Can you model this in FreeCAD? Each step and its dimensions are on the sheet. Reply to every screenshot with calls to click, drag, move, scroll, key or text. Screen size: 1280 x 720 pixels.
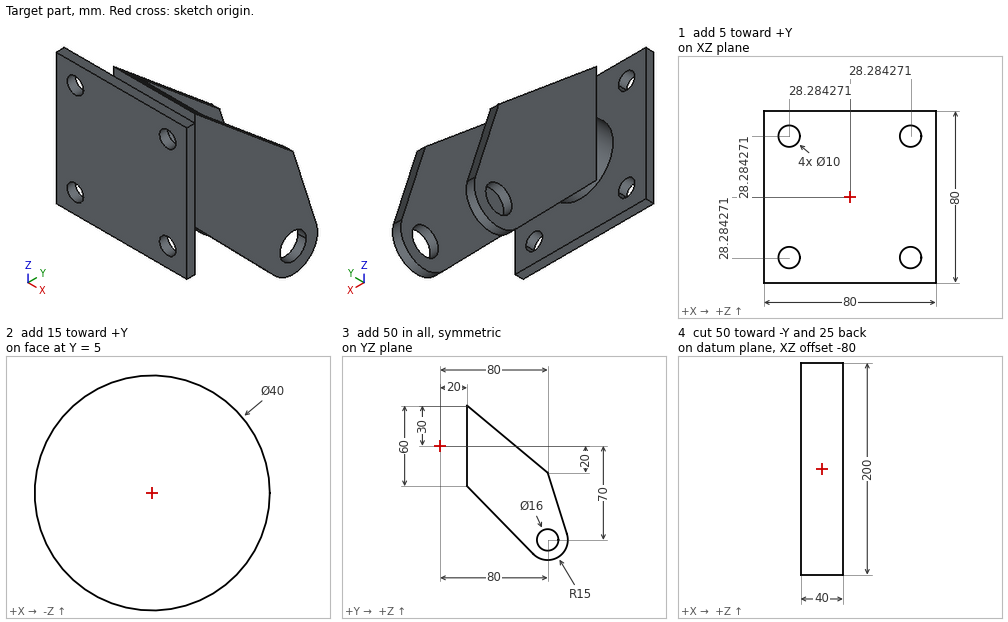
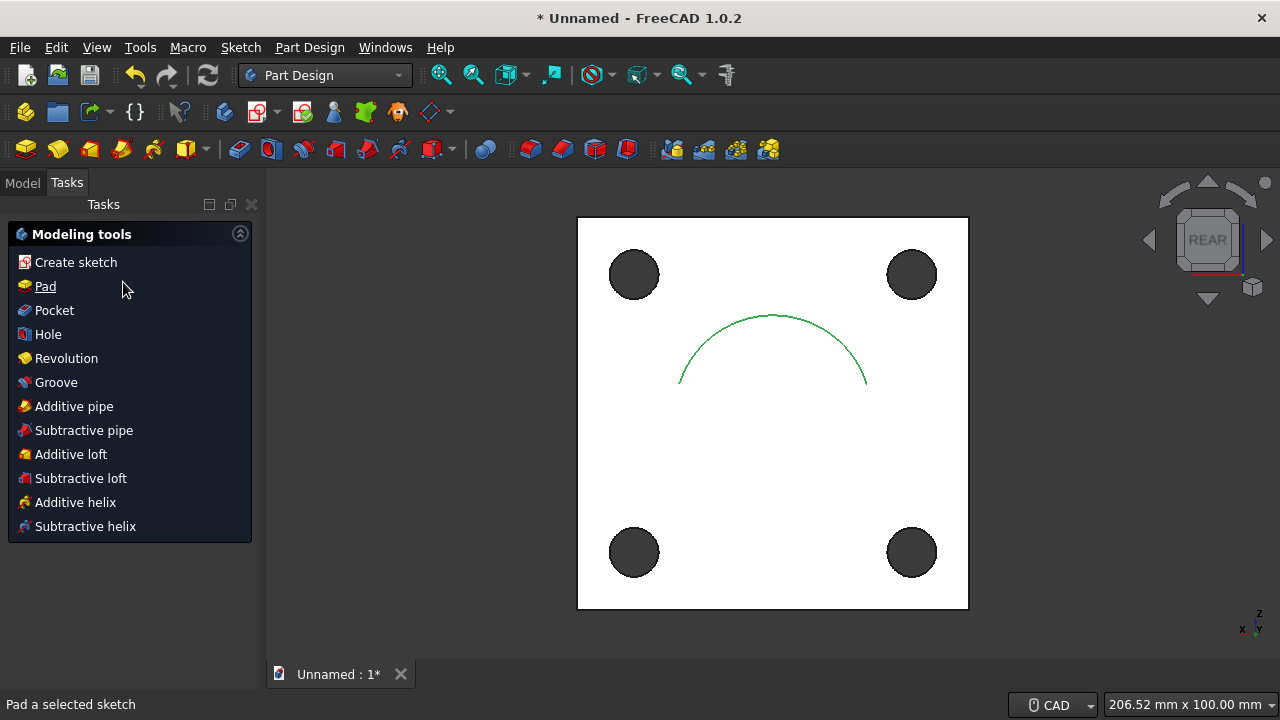
click(26, 150)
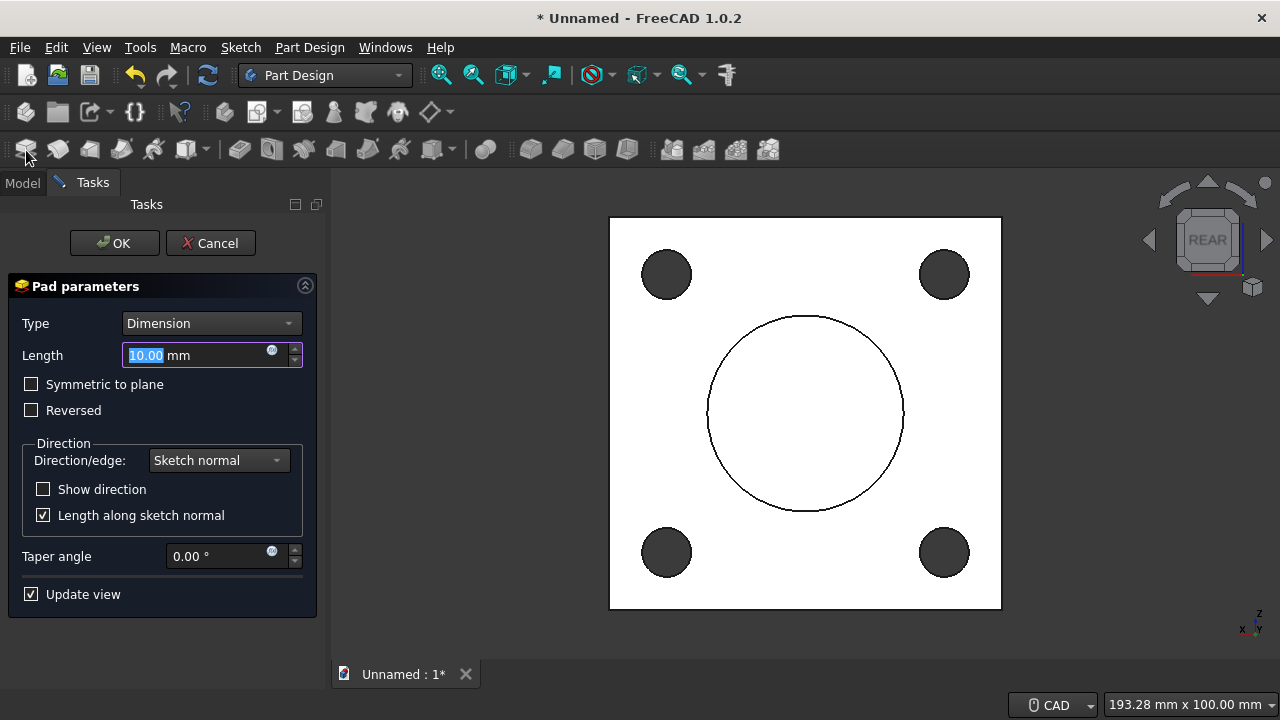
text(15)
key(Tab)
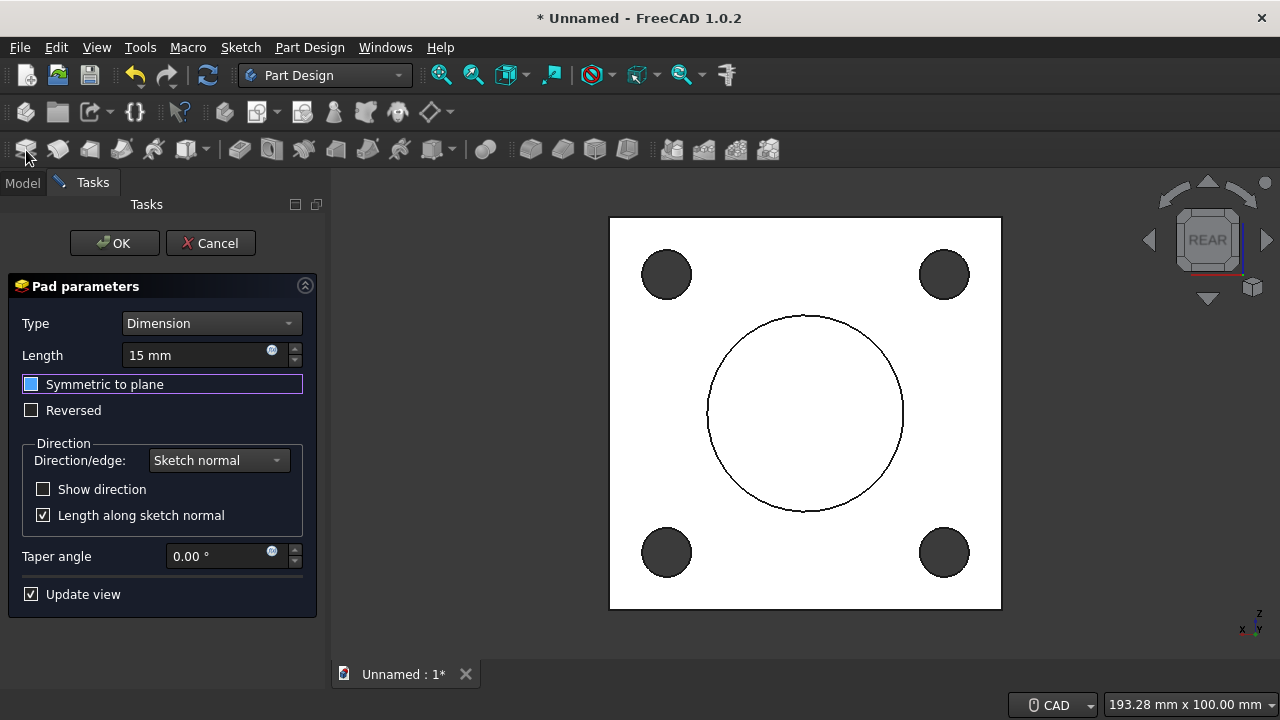
click(115, 243)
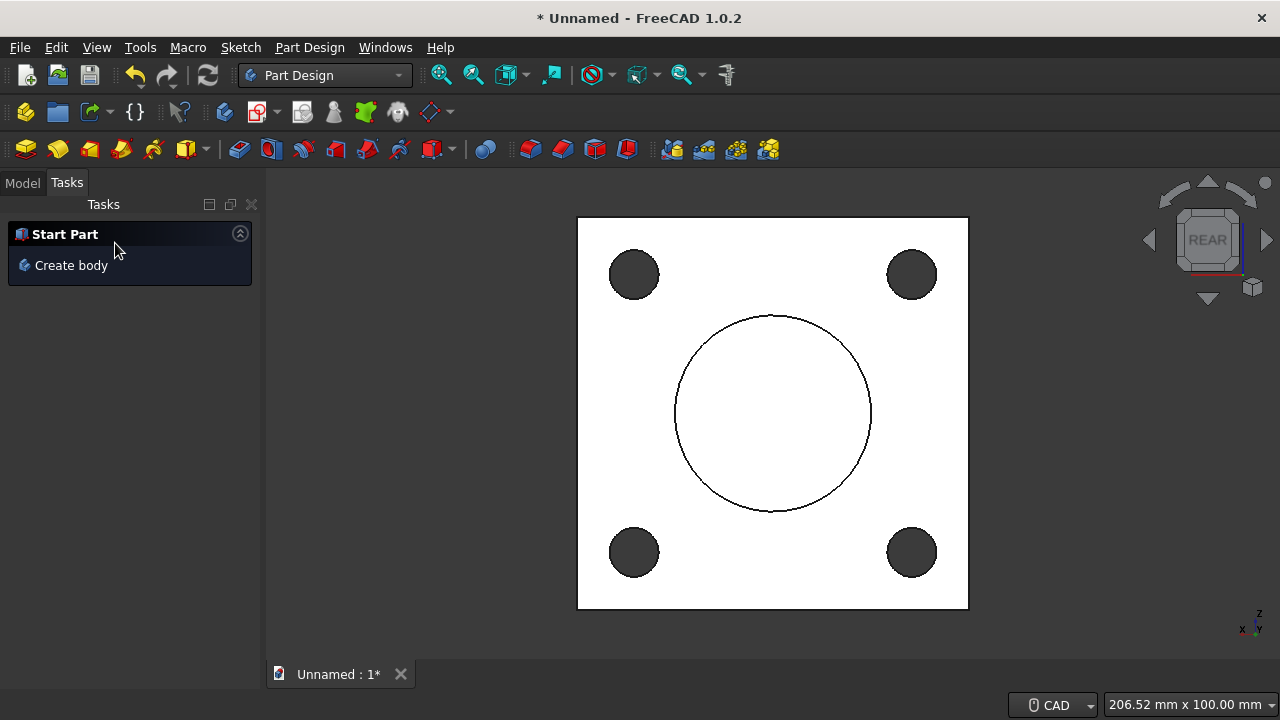
click(258, 112)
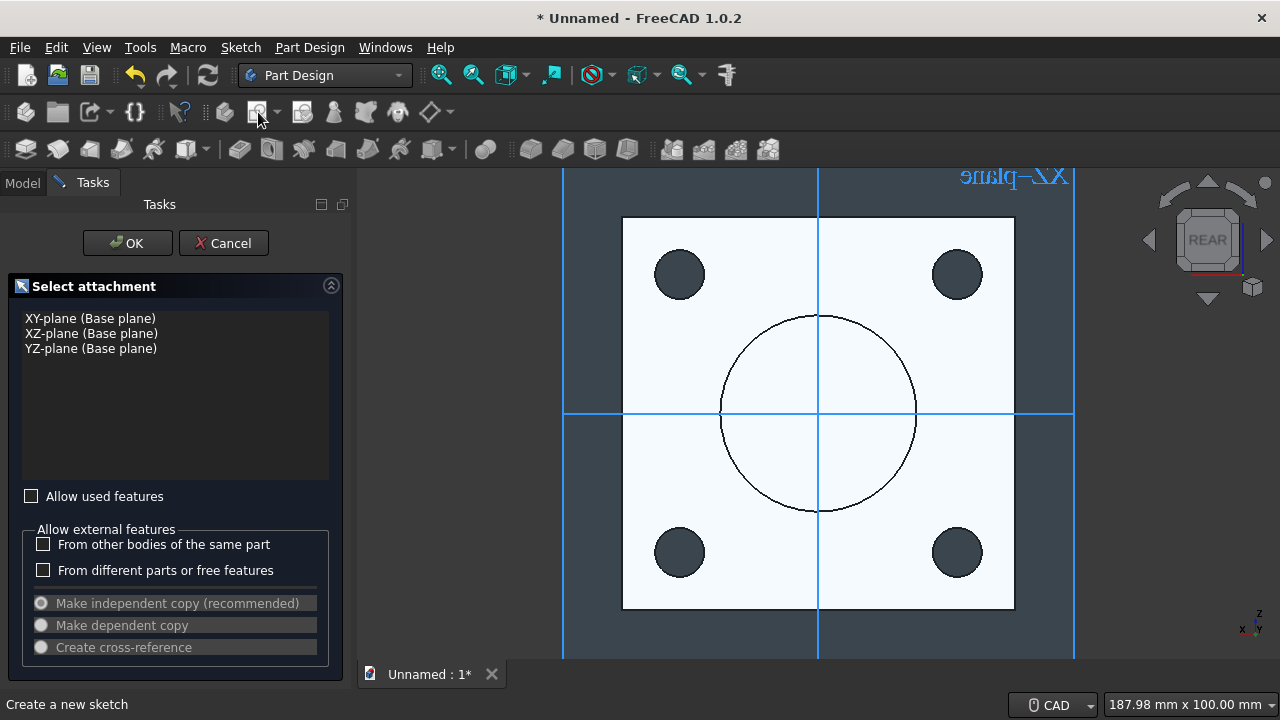
click(82, 348)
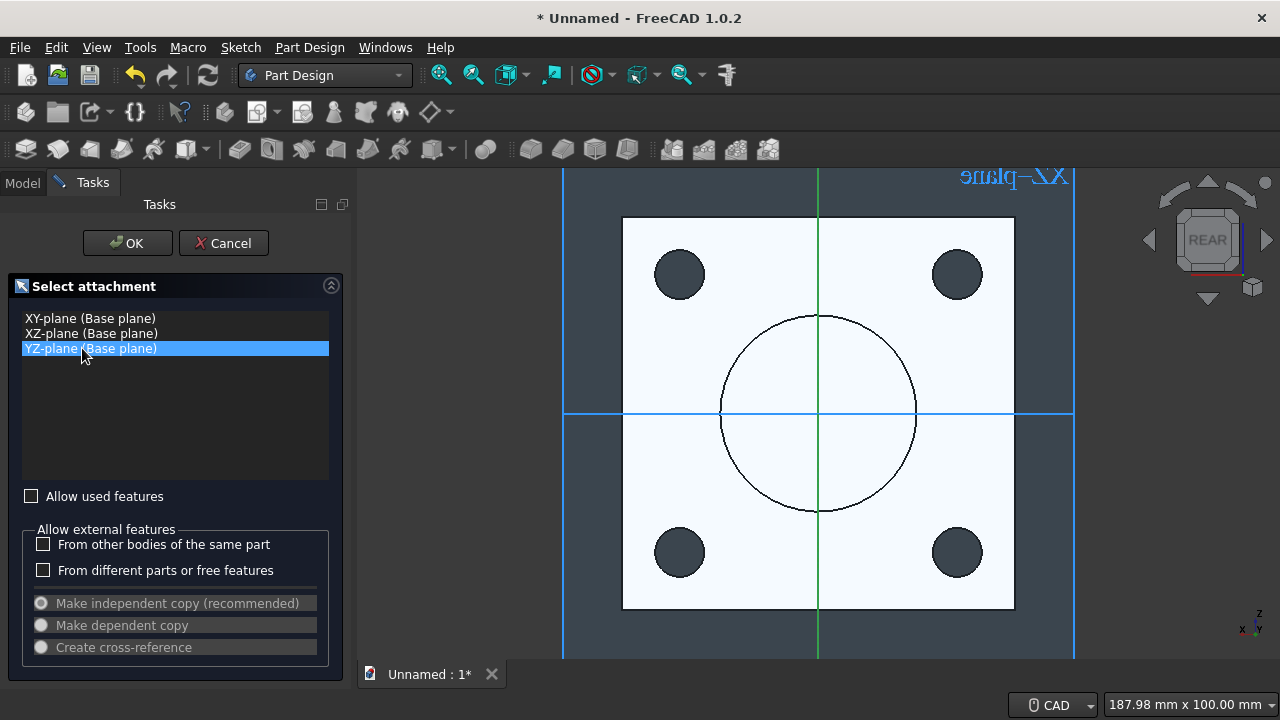
click(128, 243)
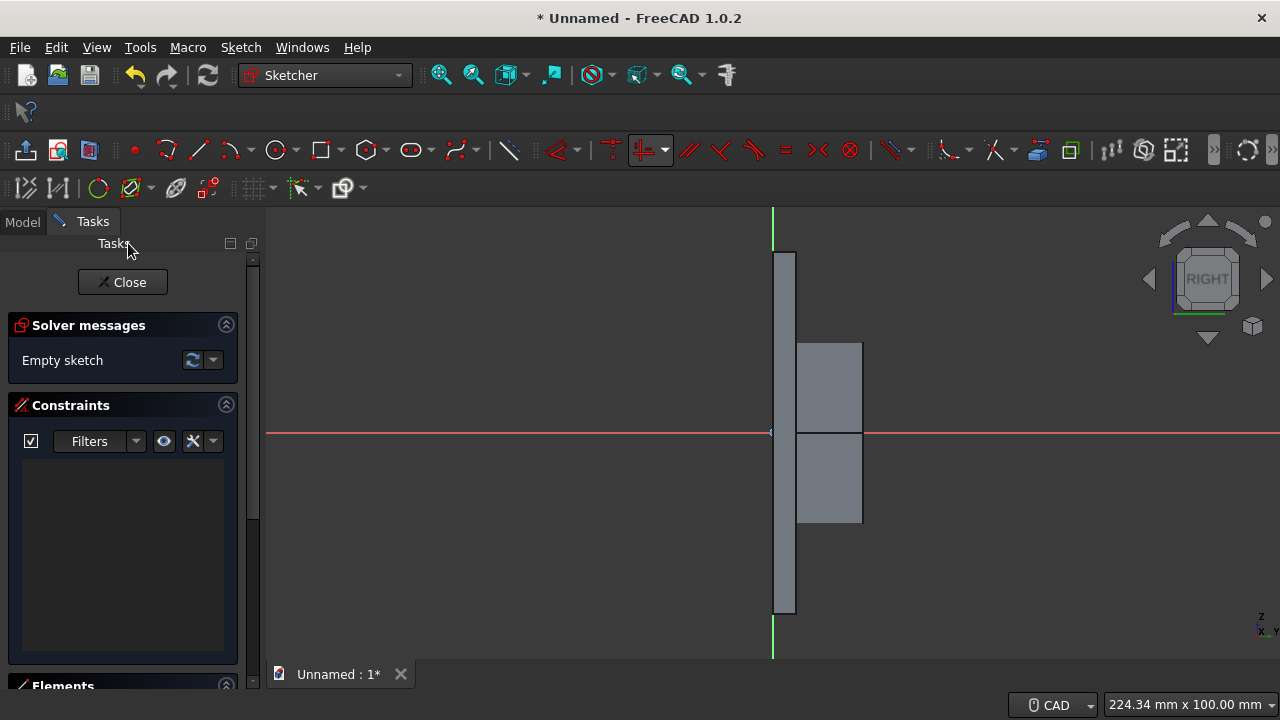
click(90, 150)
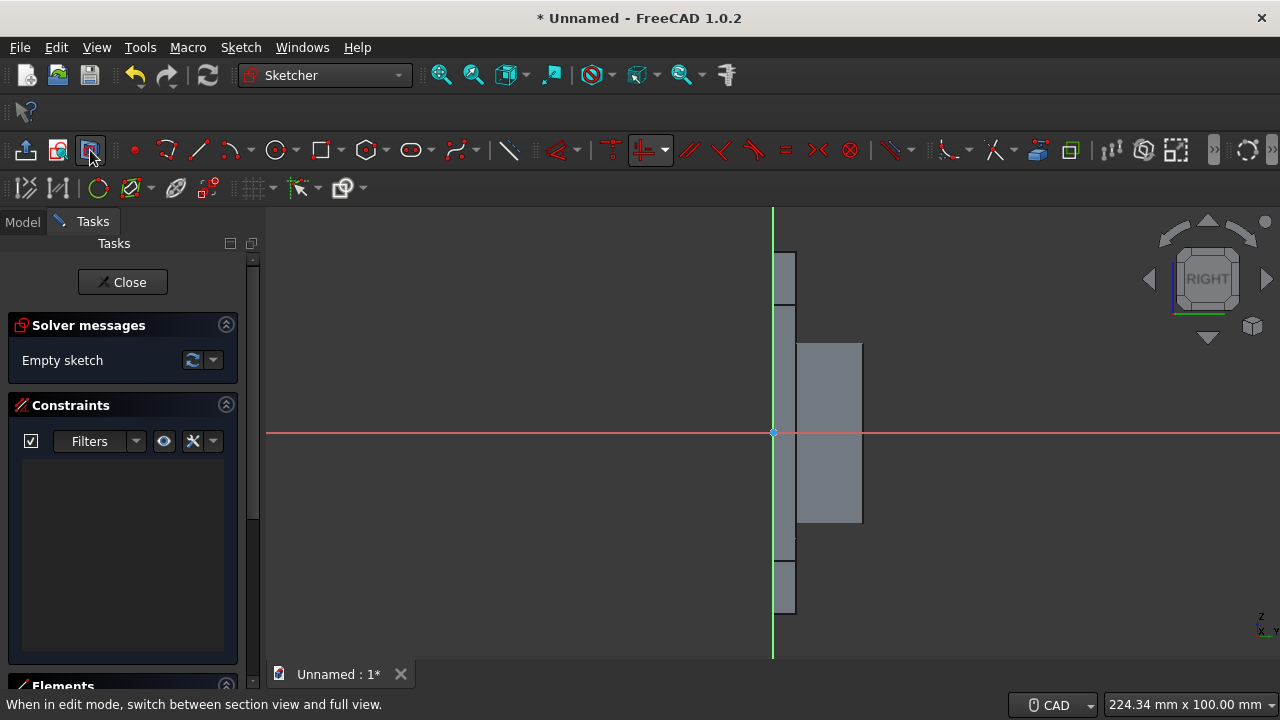
scroll(362, 288, down, 3)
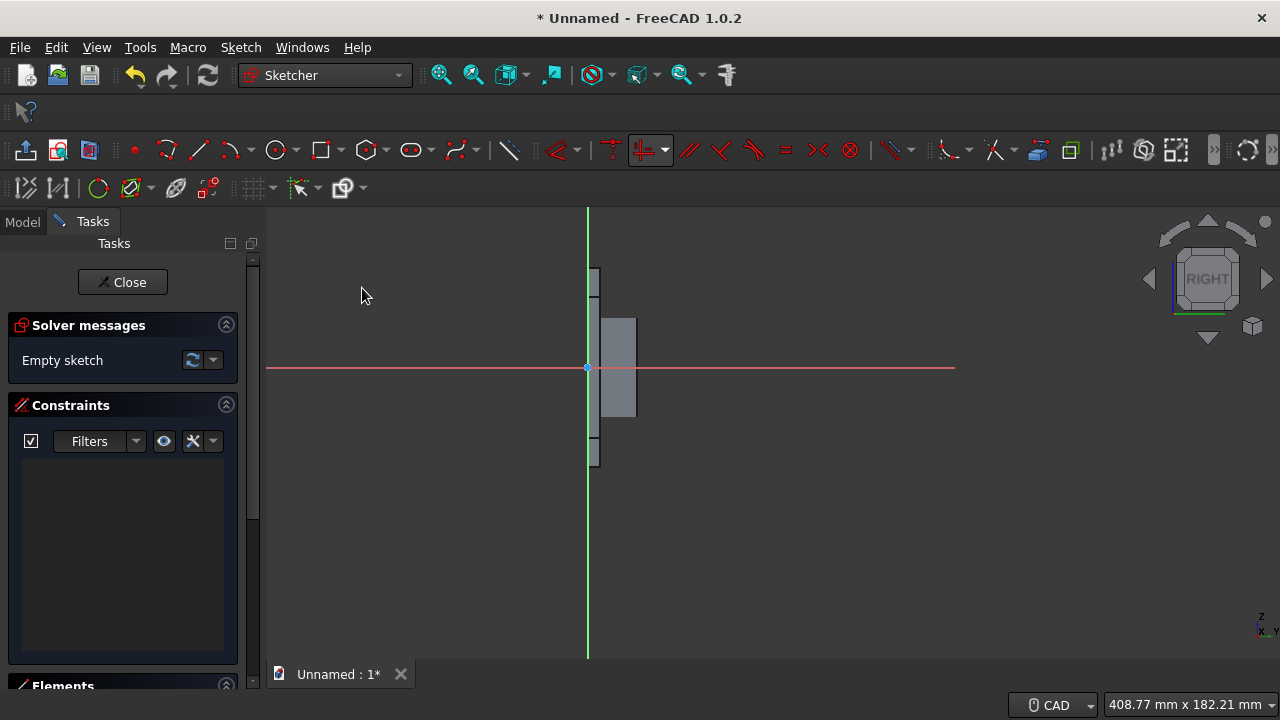
click(168, 150)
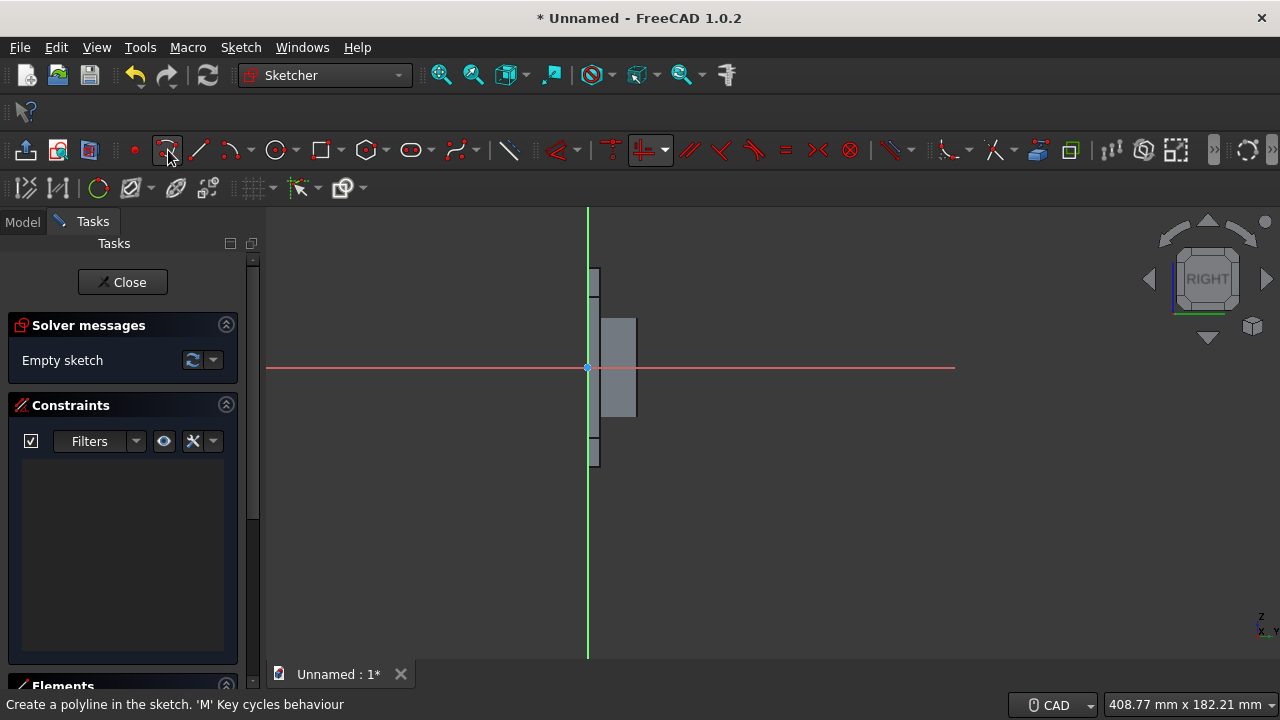
click(822, 530)
click(786, 417)
click(637, 293)
click(637, 442)
click(759, 567)
right_click(759, 567)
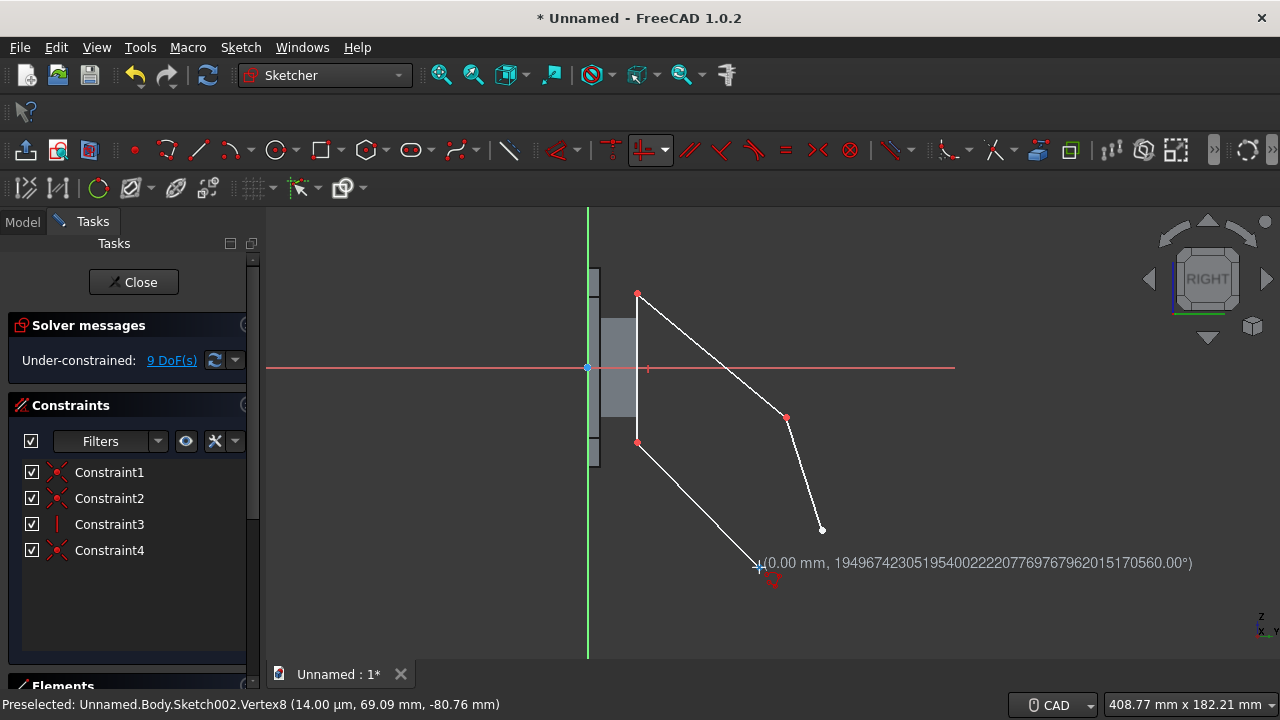
click(254, 150)